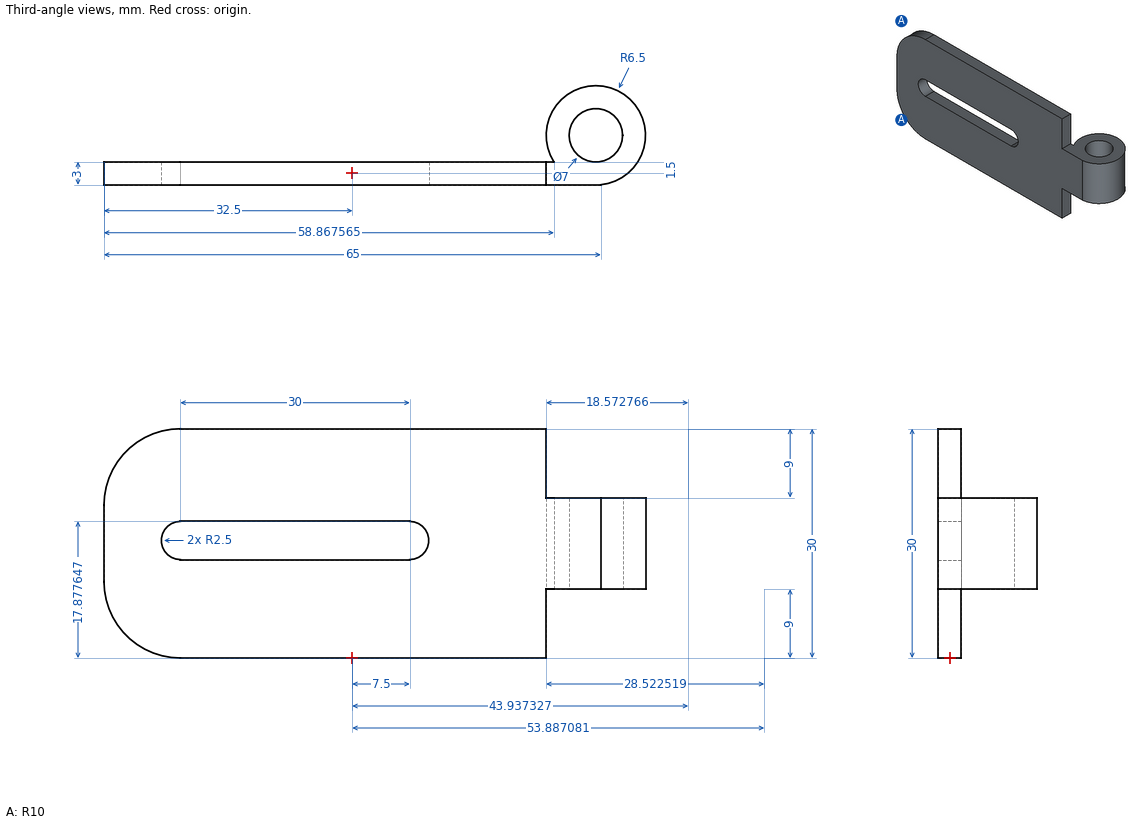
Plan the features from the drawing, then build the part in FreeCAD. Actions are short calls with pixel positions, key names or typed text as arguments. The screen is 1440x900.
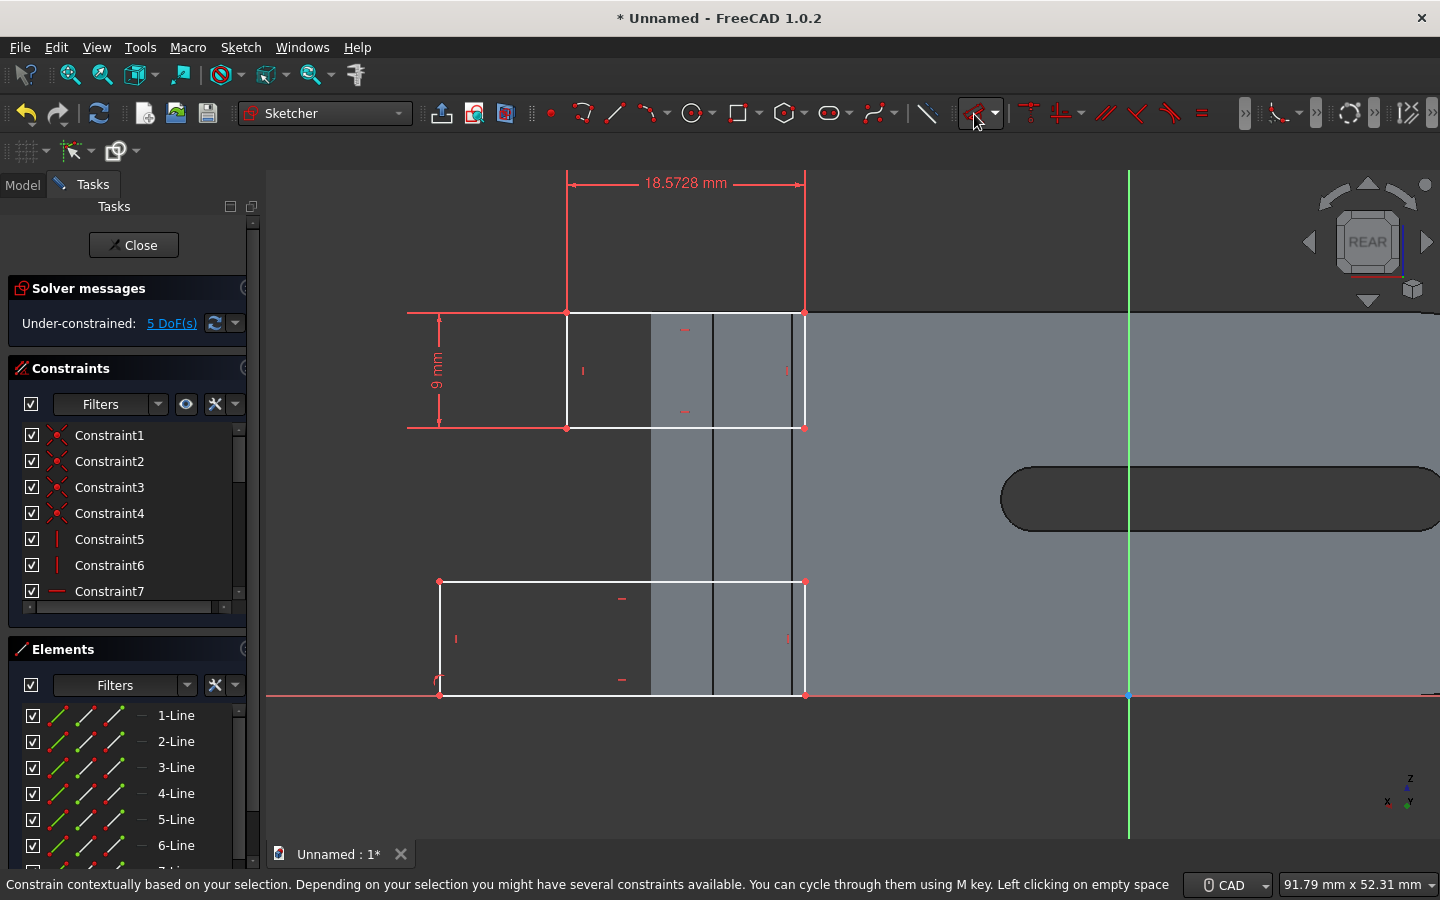
click(440, 616)
click(406, 639)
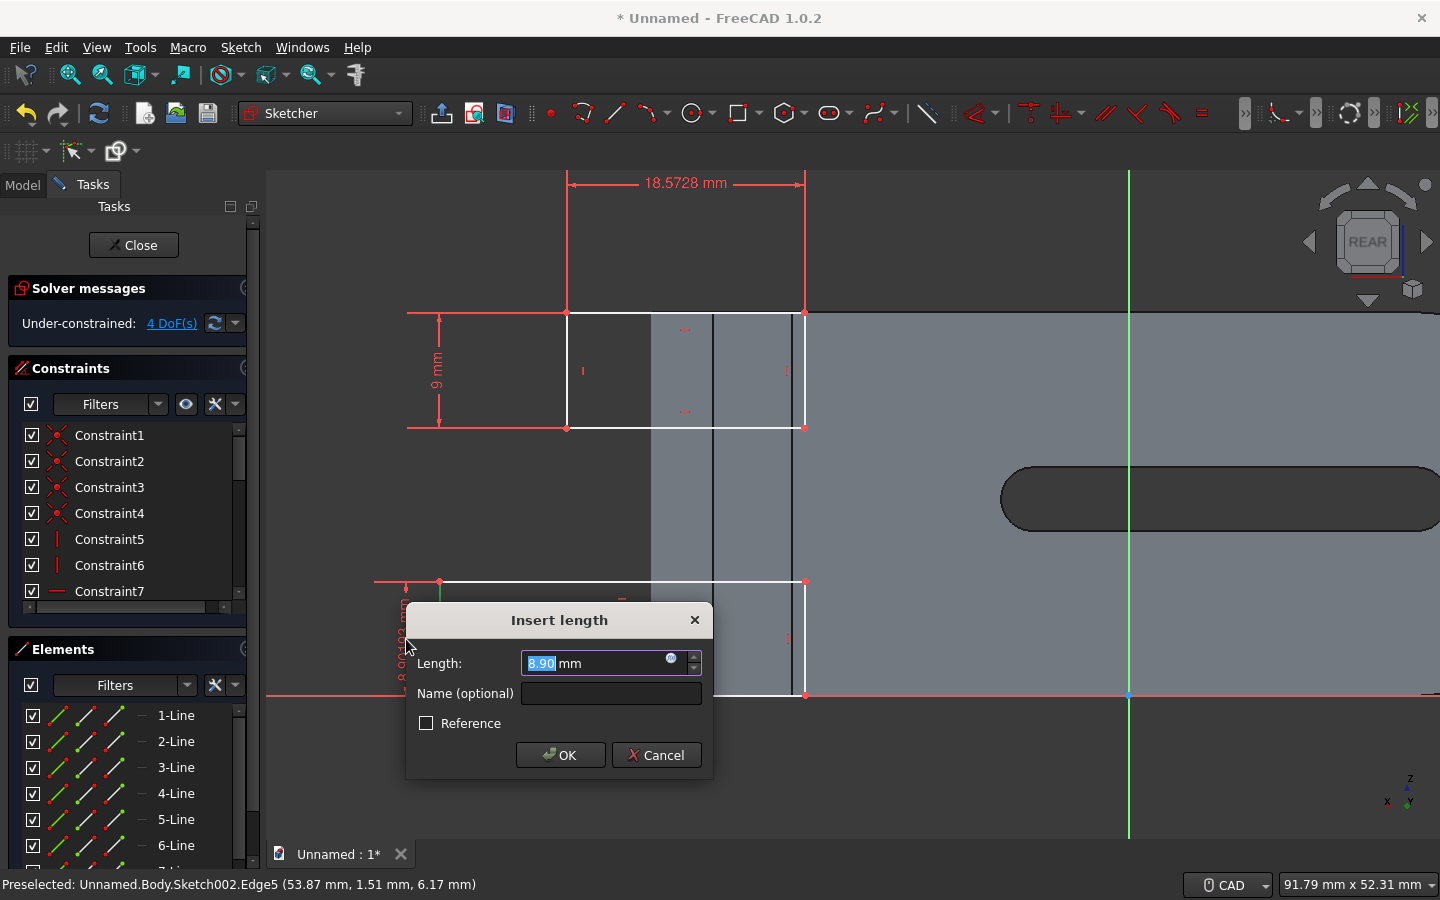
text(9)
key(Return)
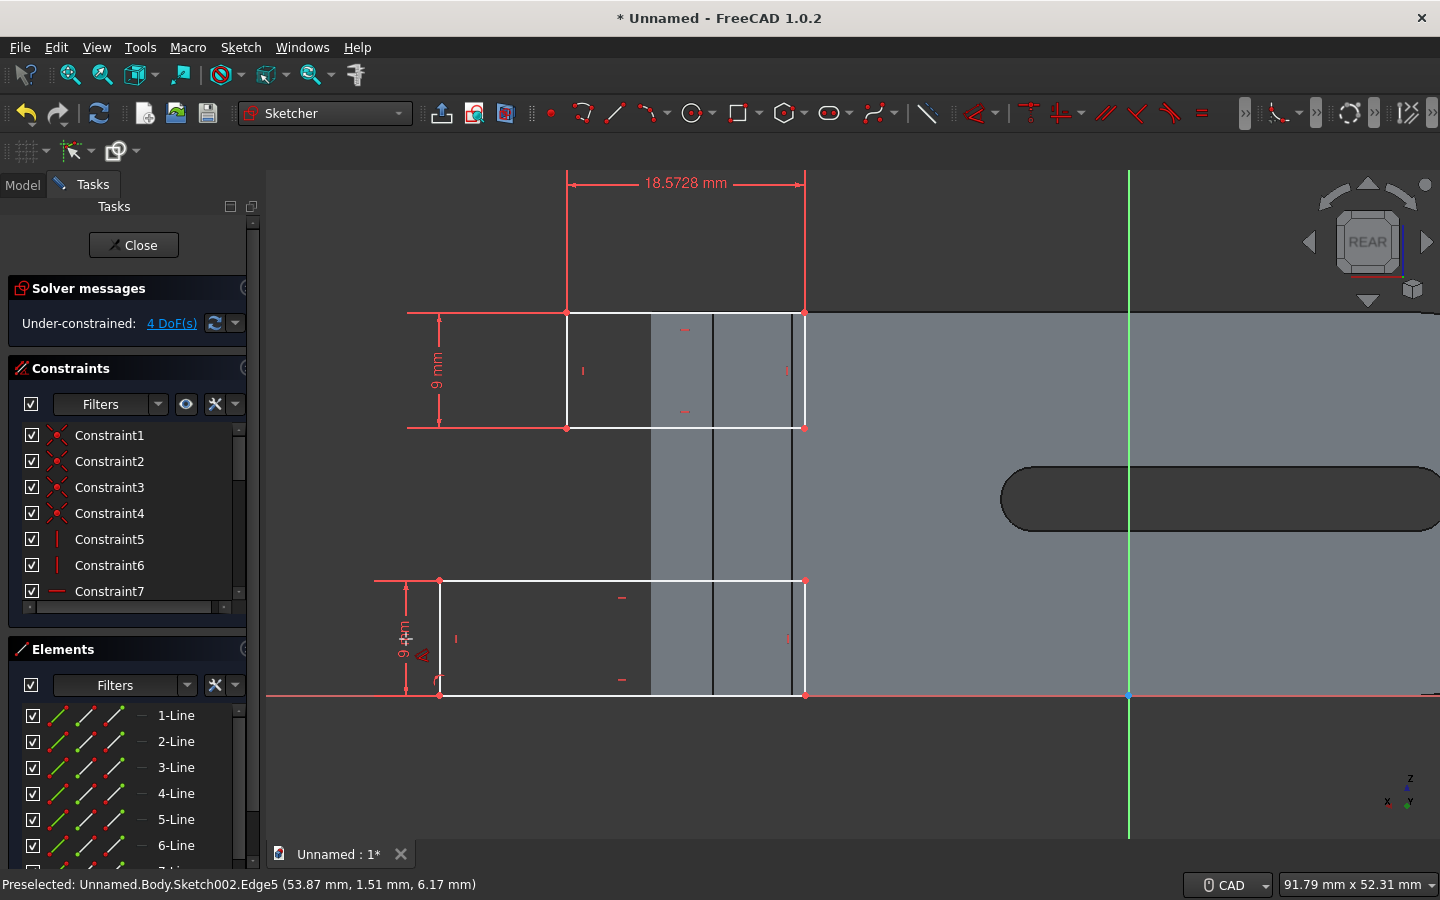
click(567, 313)
click(1163, 504)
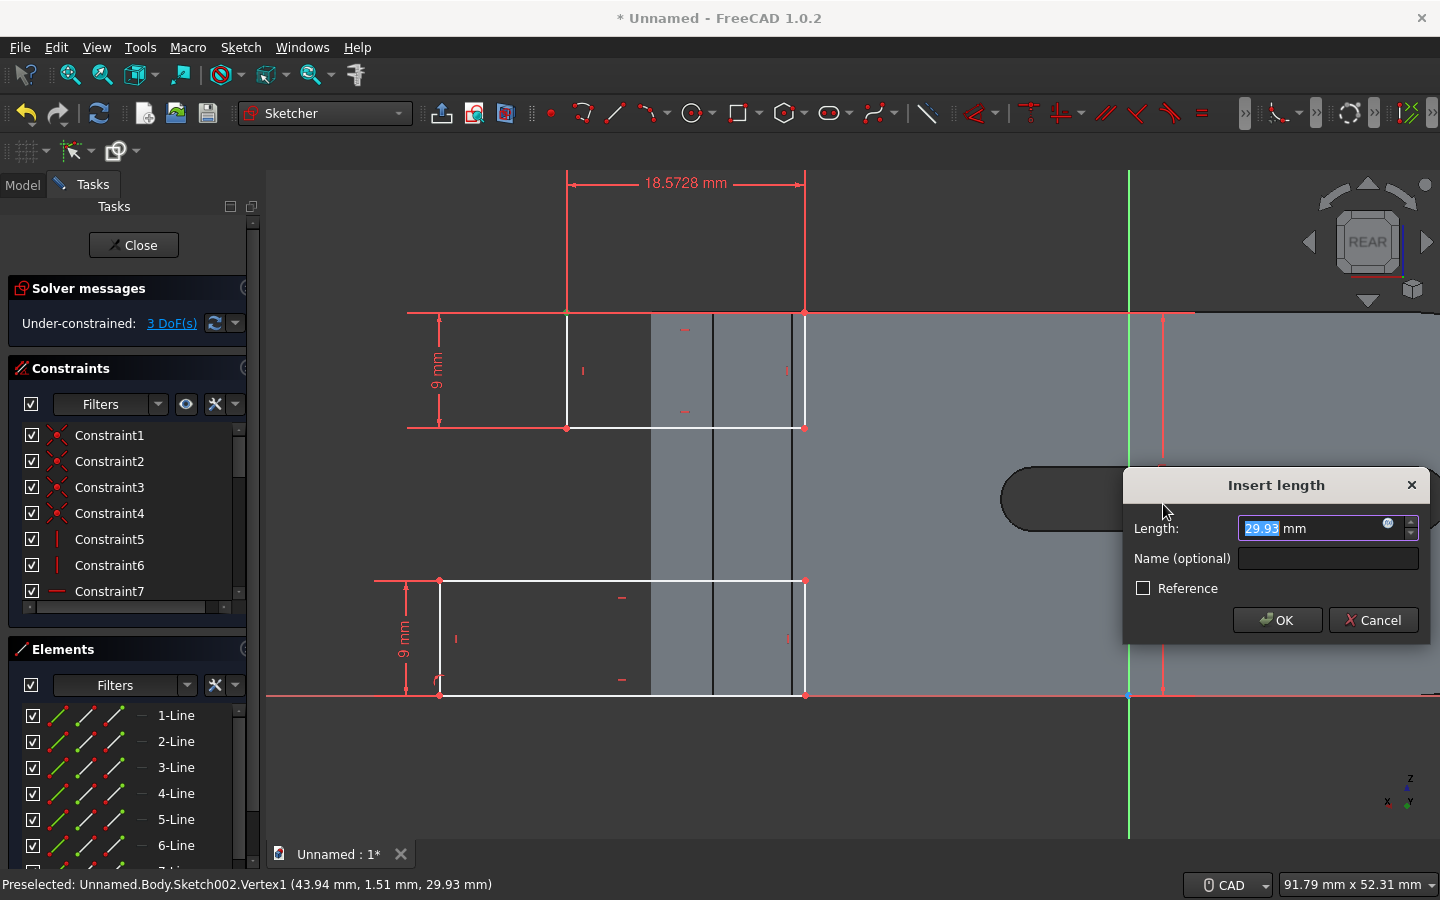
text(30)
key(Return)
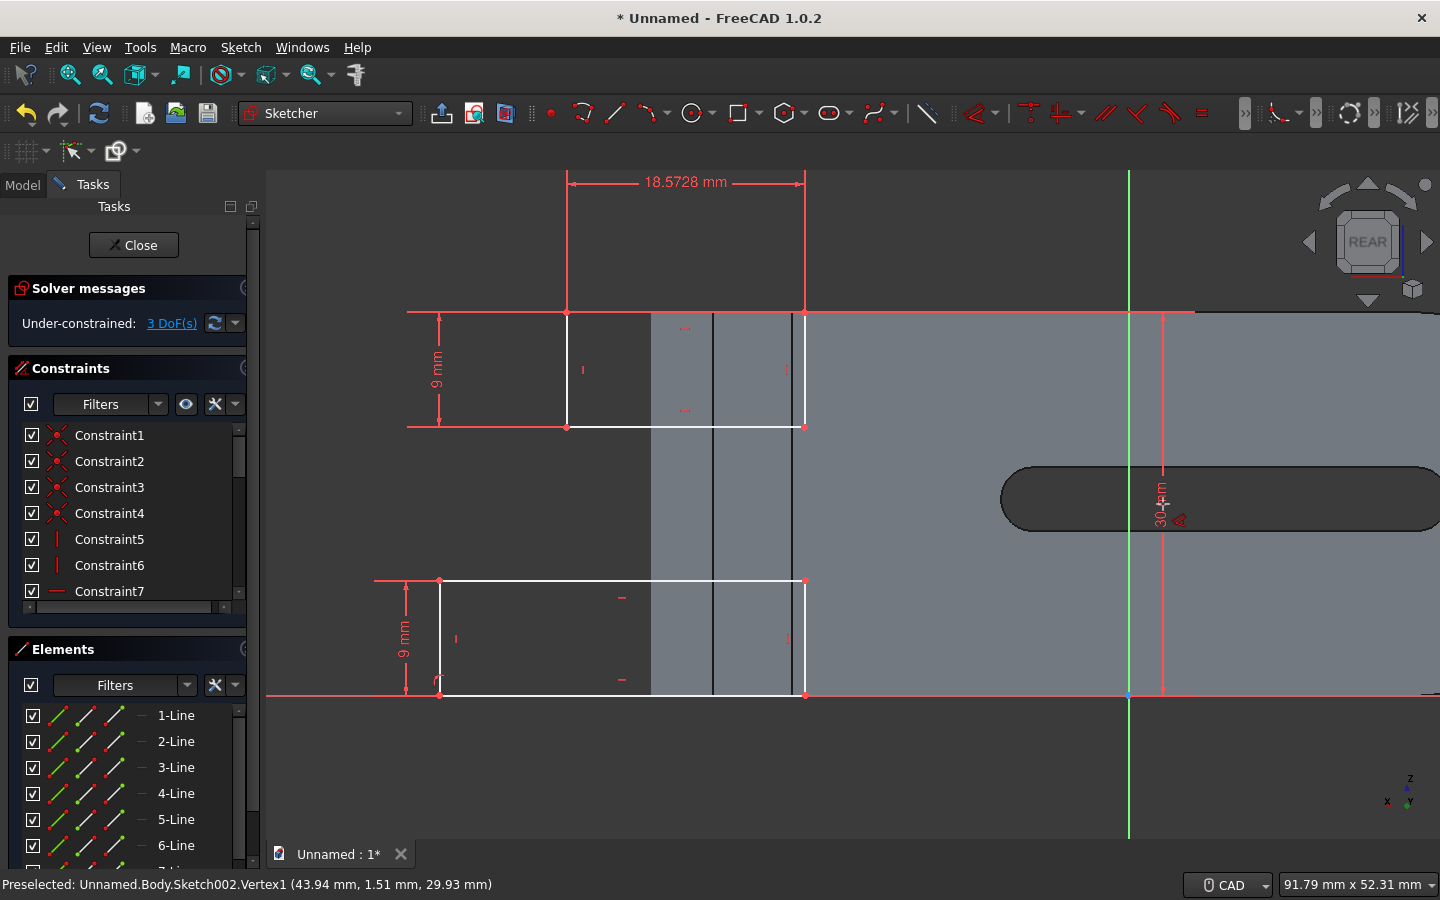
click(550, 696)
click(623, 730)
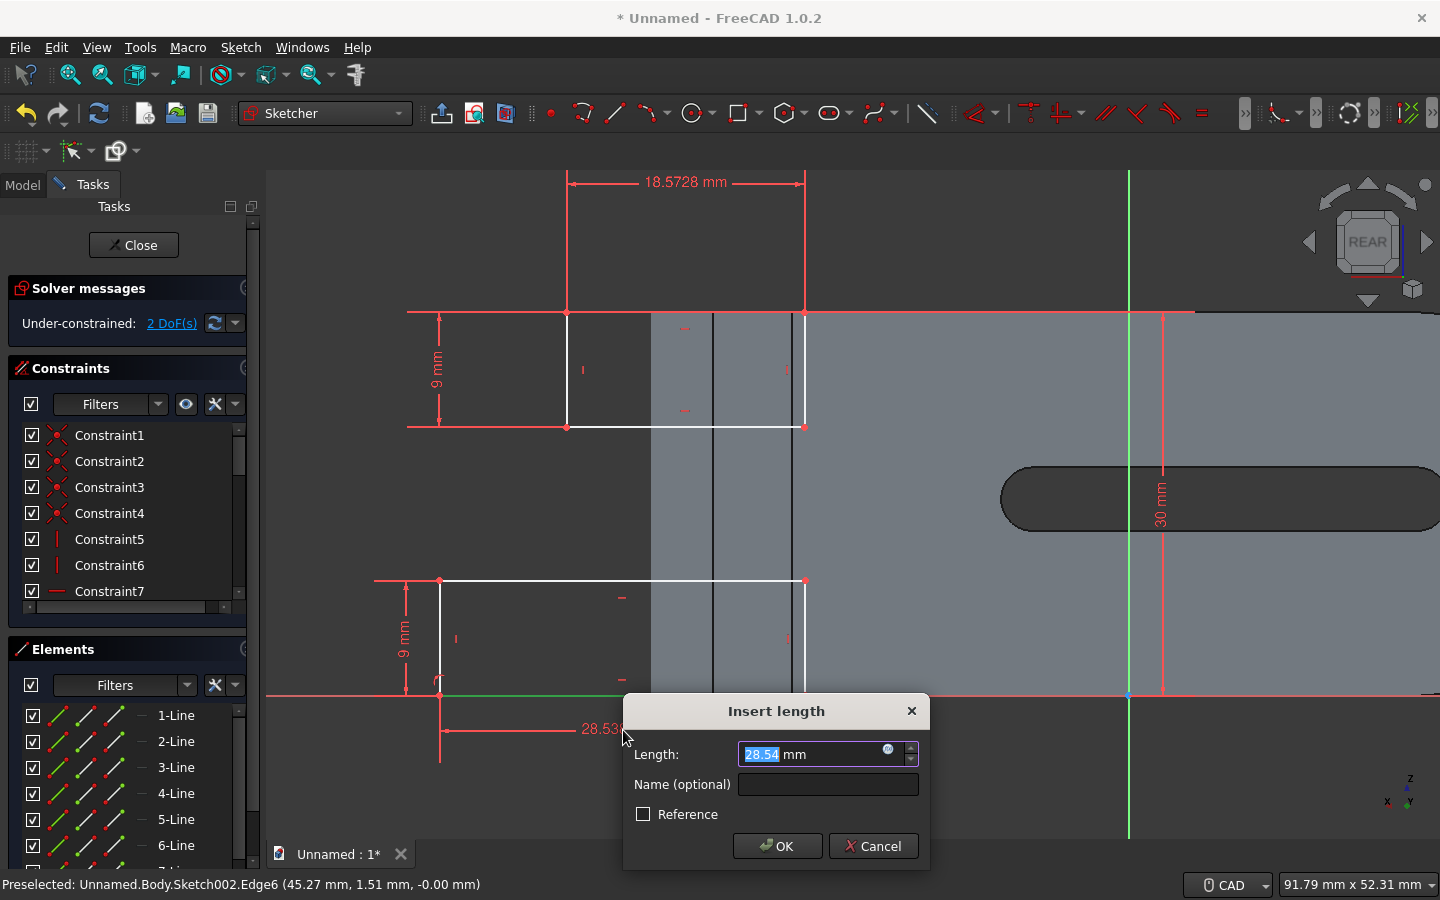
text(28.522519)
key(Return)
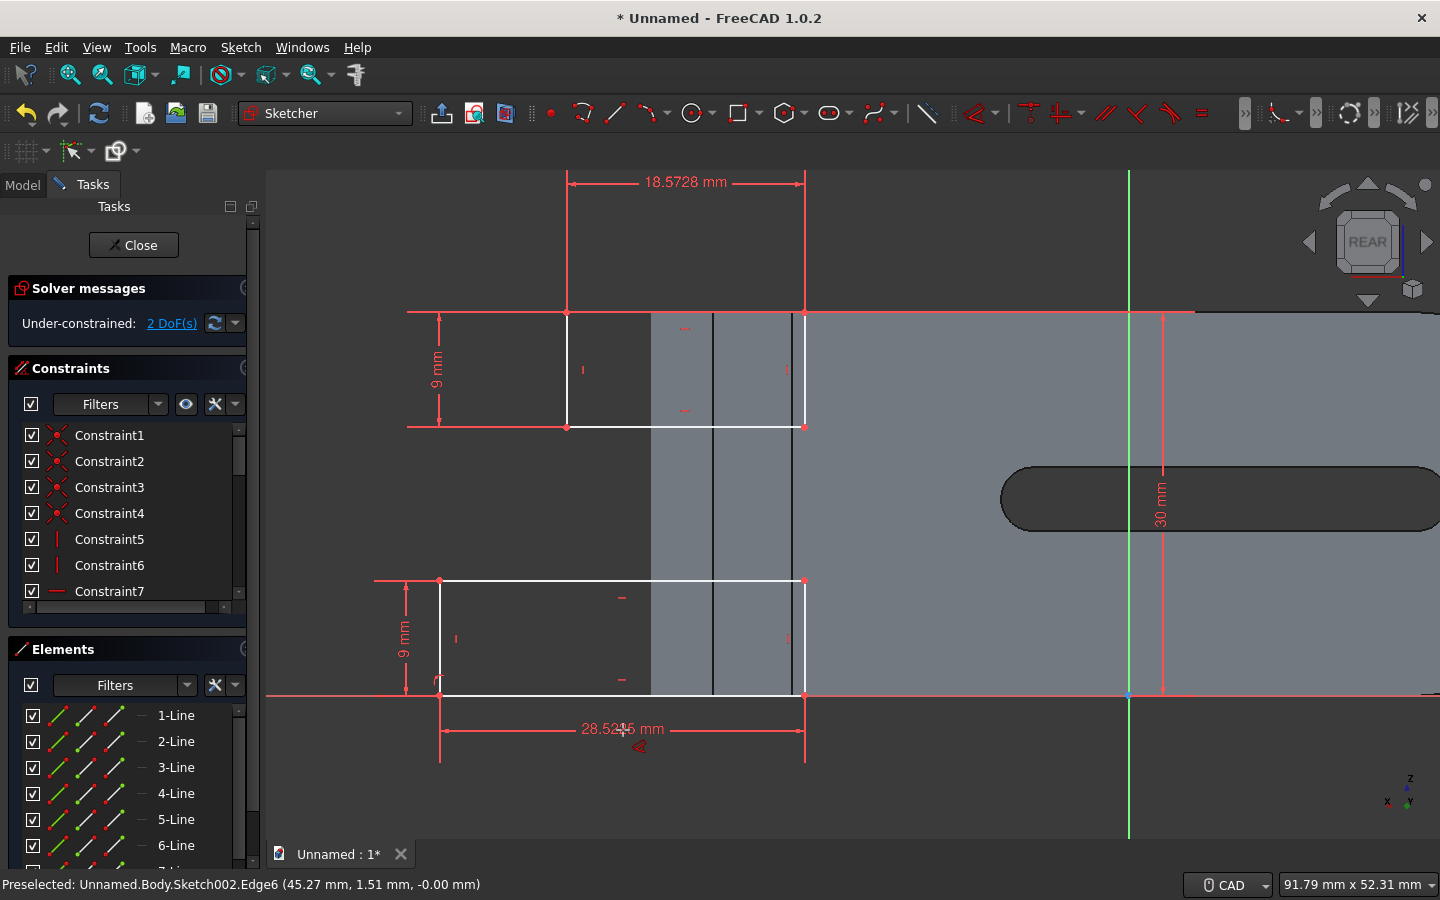
click(567, 312)
click(848, 730)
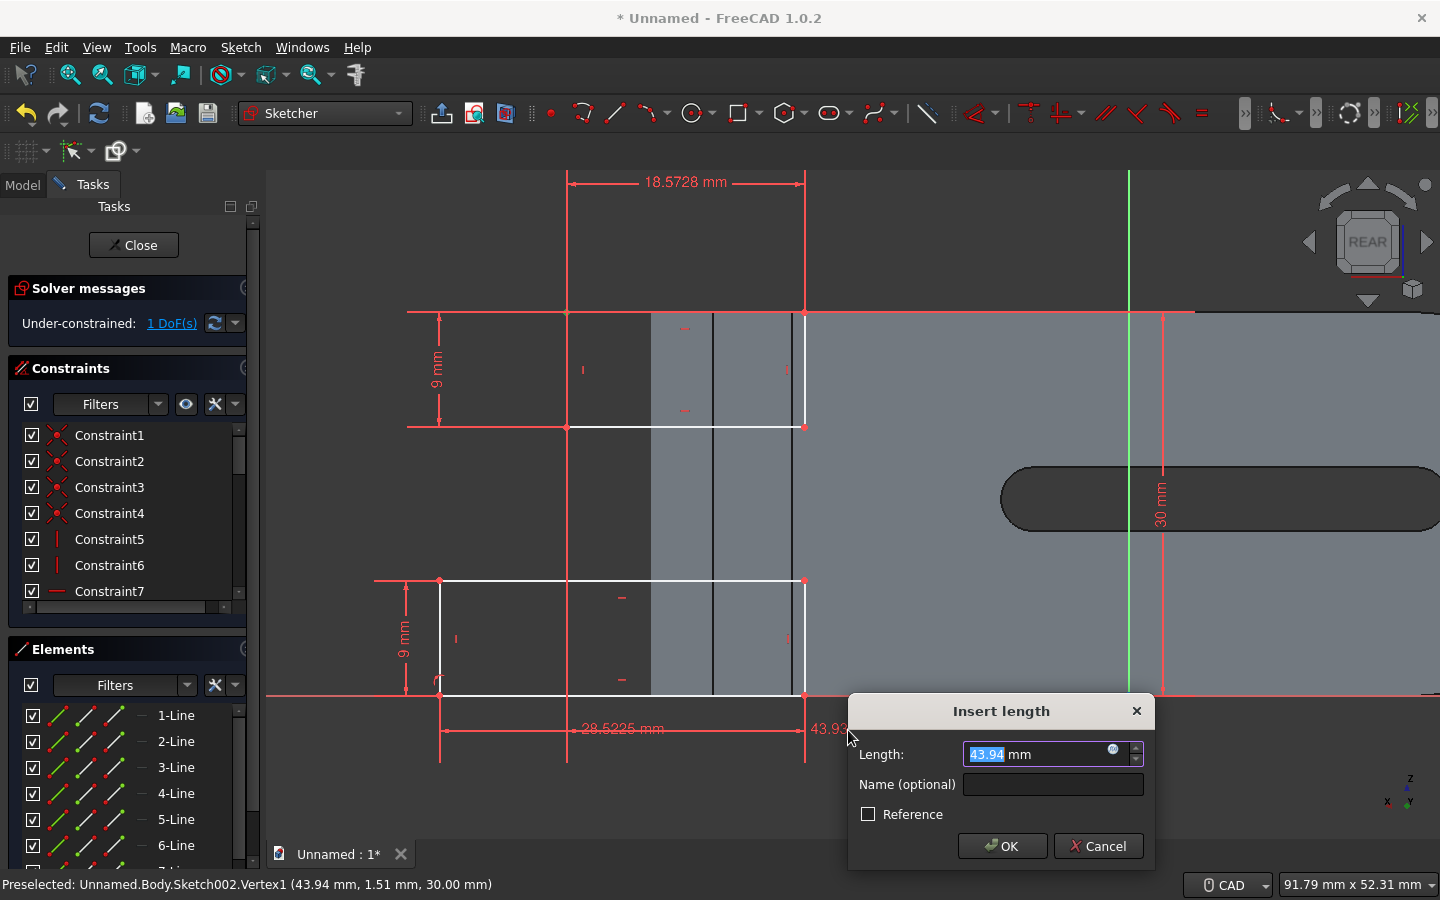
text(43.937327)
key(Return)